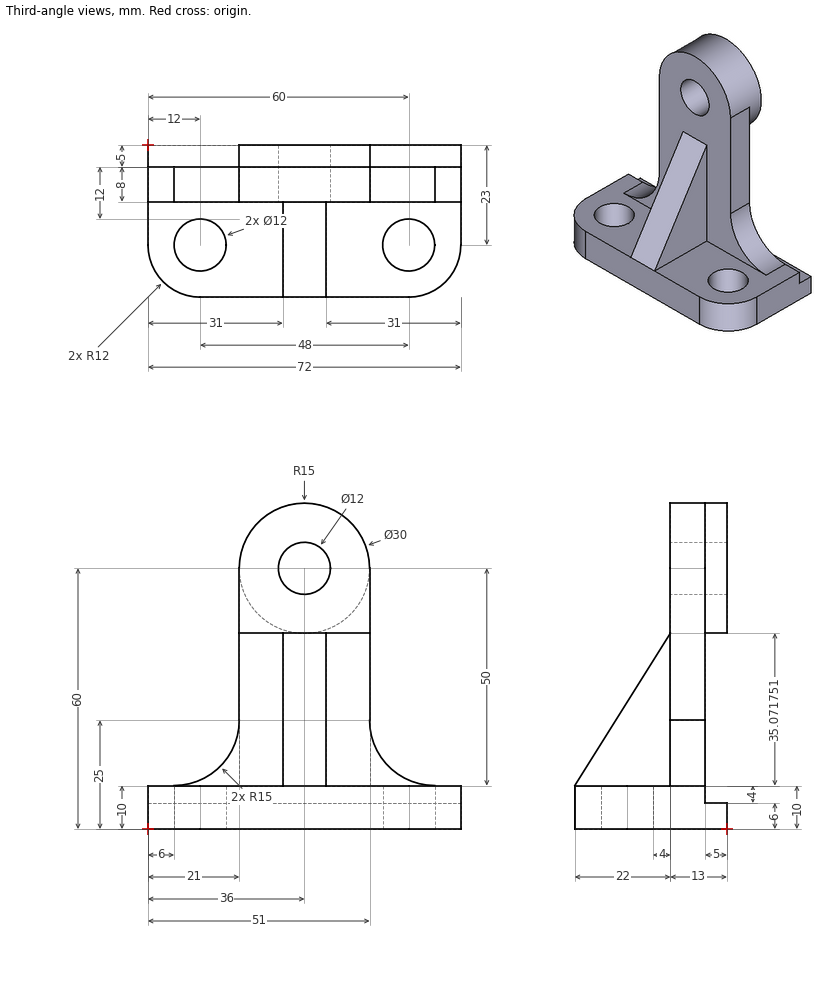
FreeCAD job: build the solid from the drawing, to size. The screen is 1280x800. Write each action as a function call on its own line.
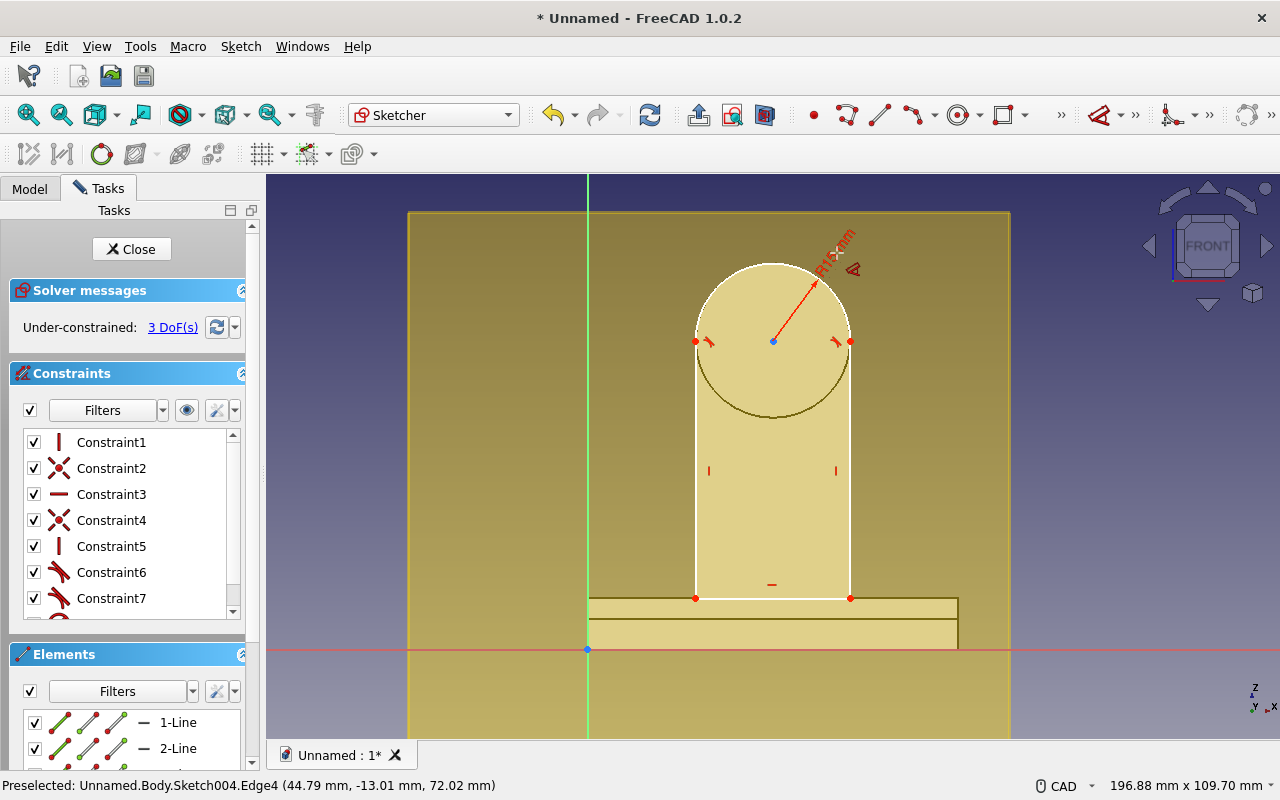
click(696, 418)
click(662, 470)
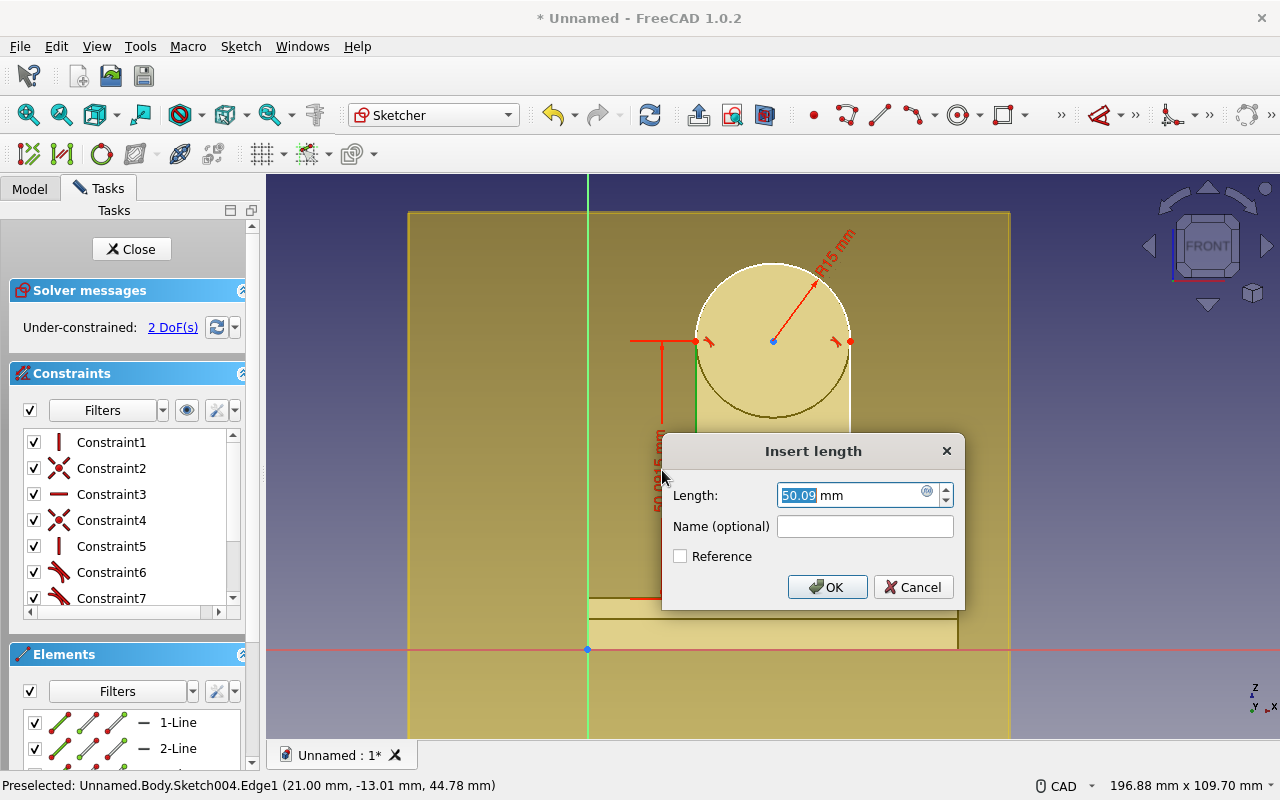
text(50)
key(Return)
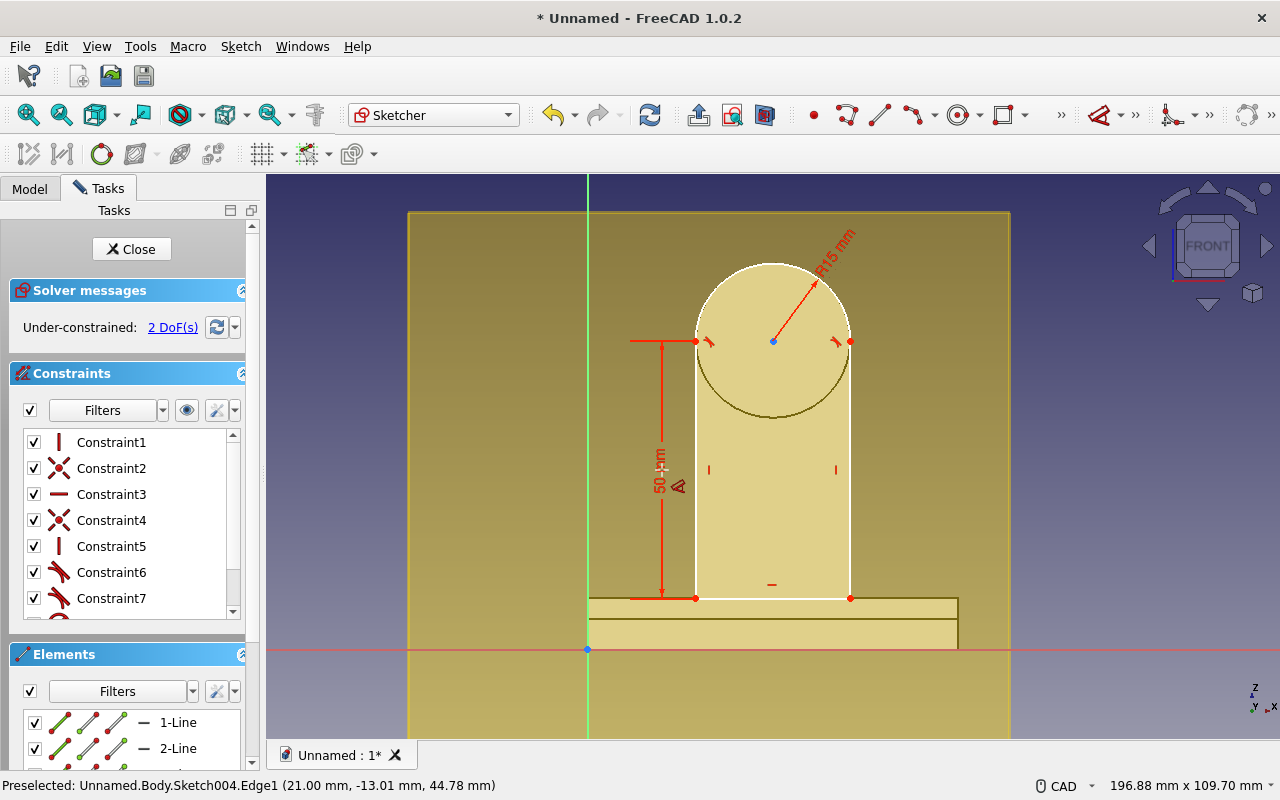
click(696, 341)
click(642, 684)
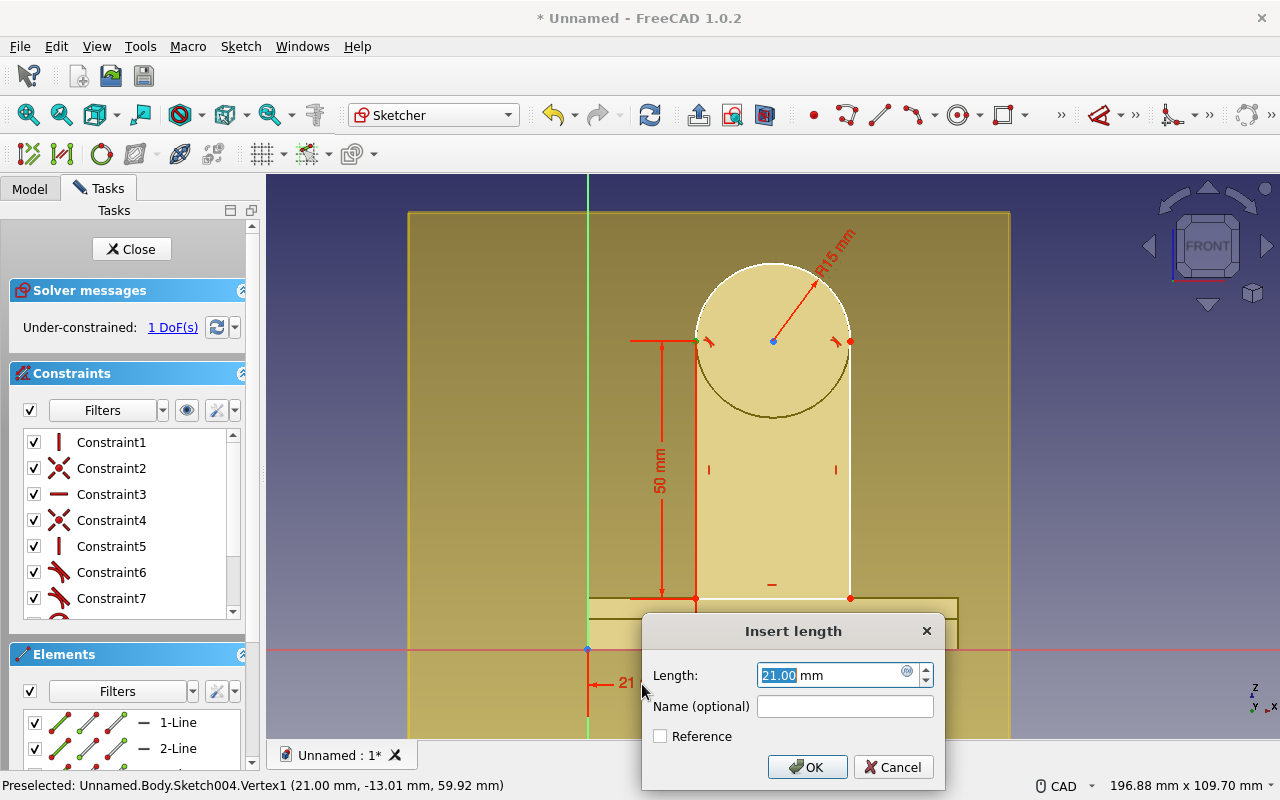
text(21)
key(Return)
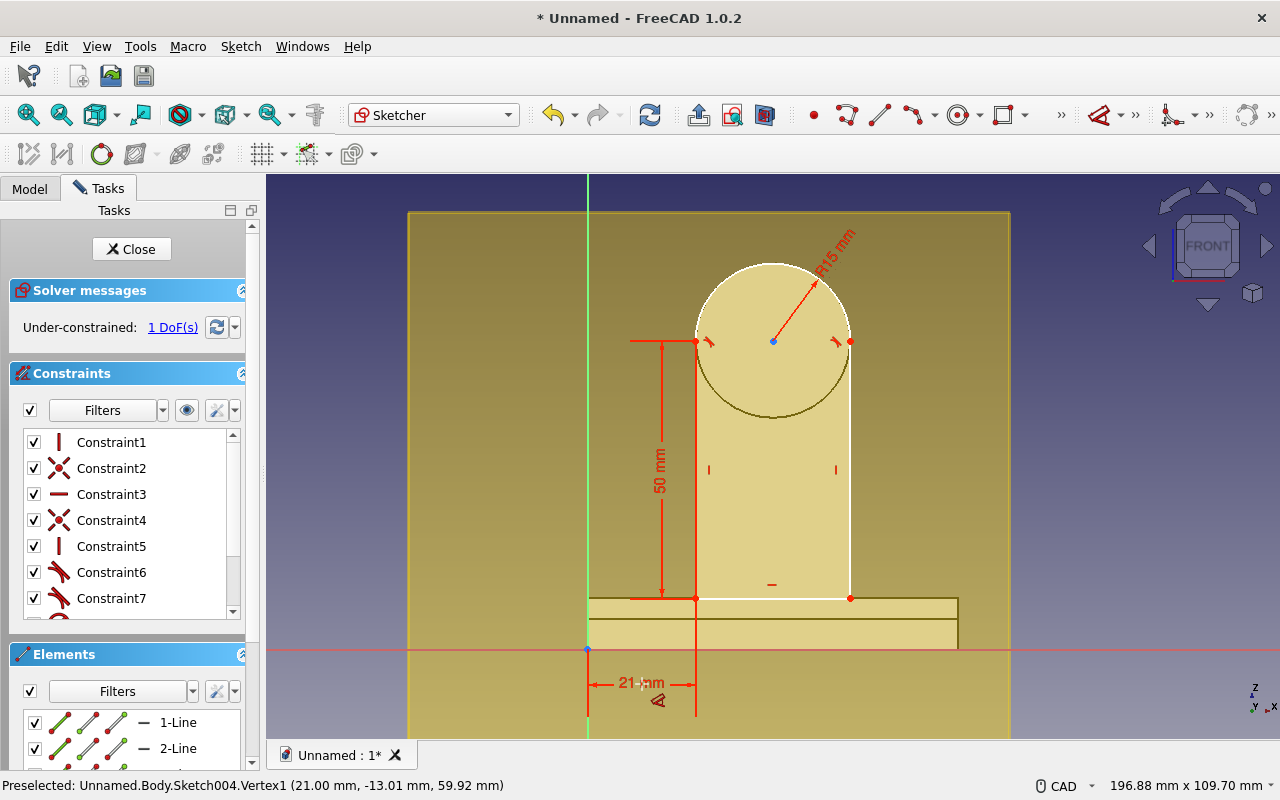
click(696, 341)
click(554, 495)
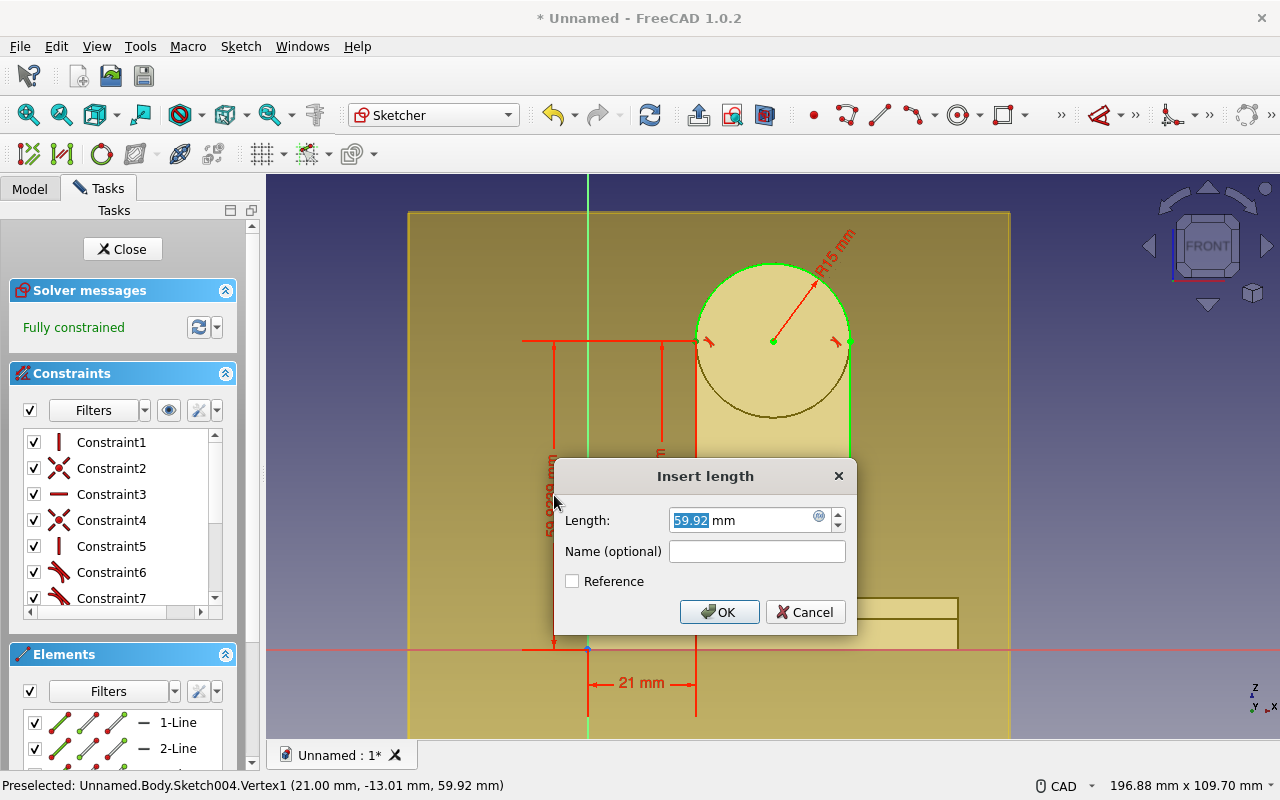
text(60)
key(Return)
key(Escape)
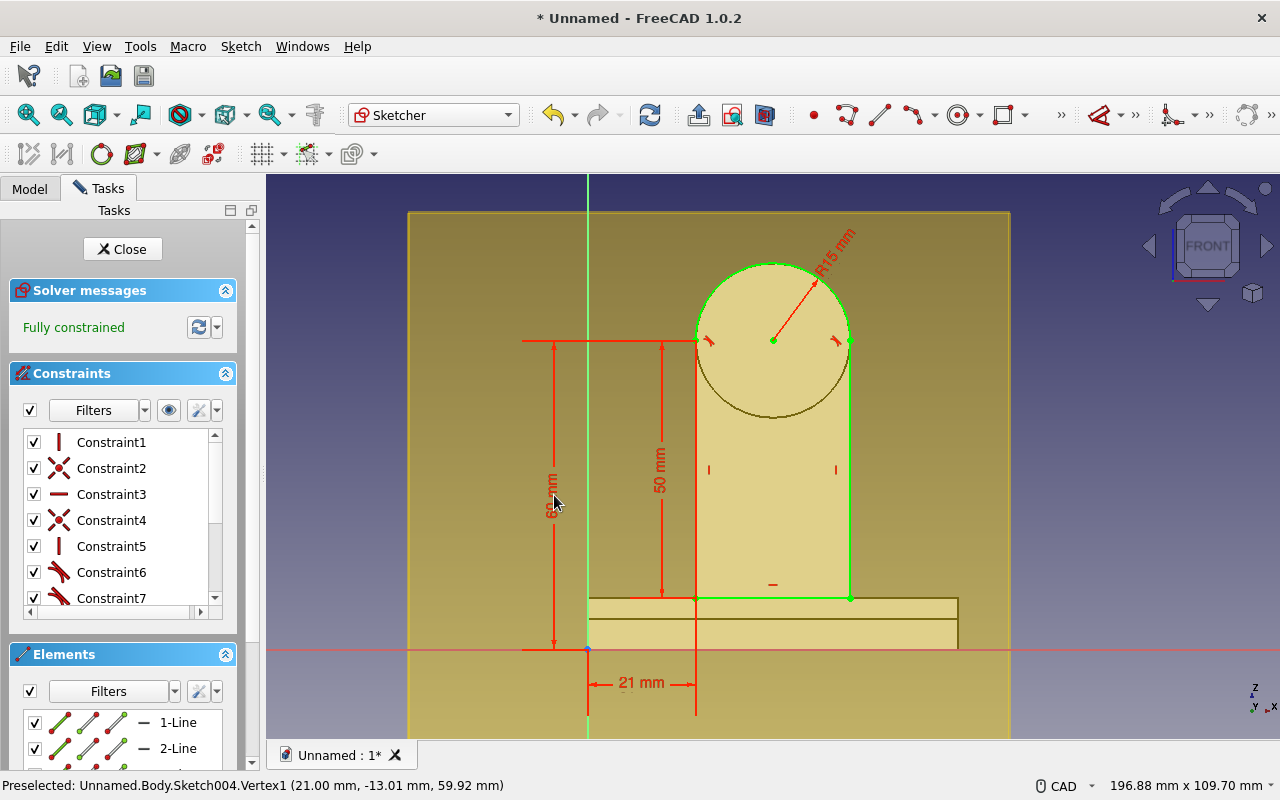
click(123, 249)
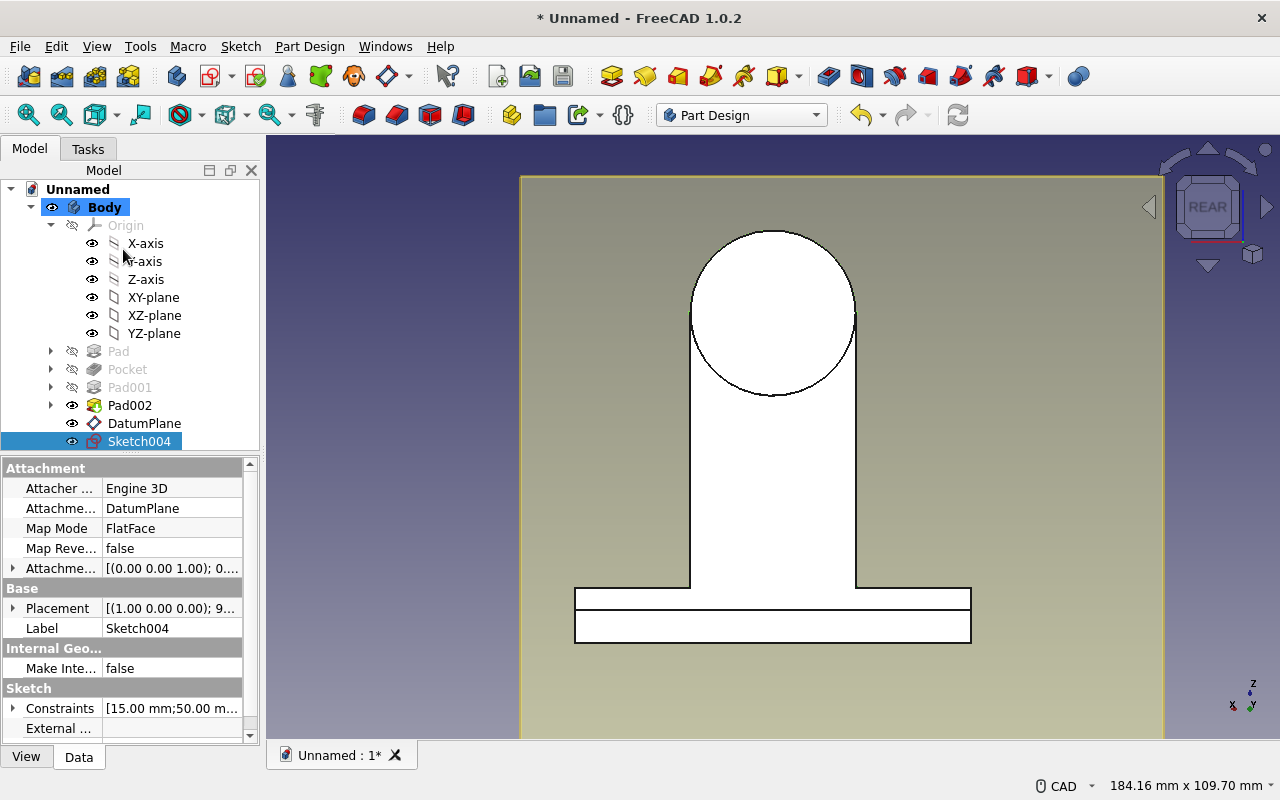
click(829, 76)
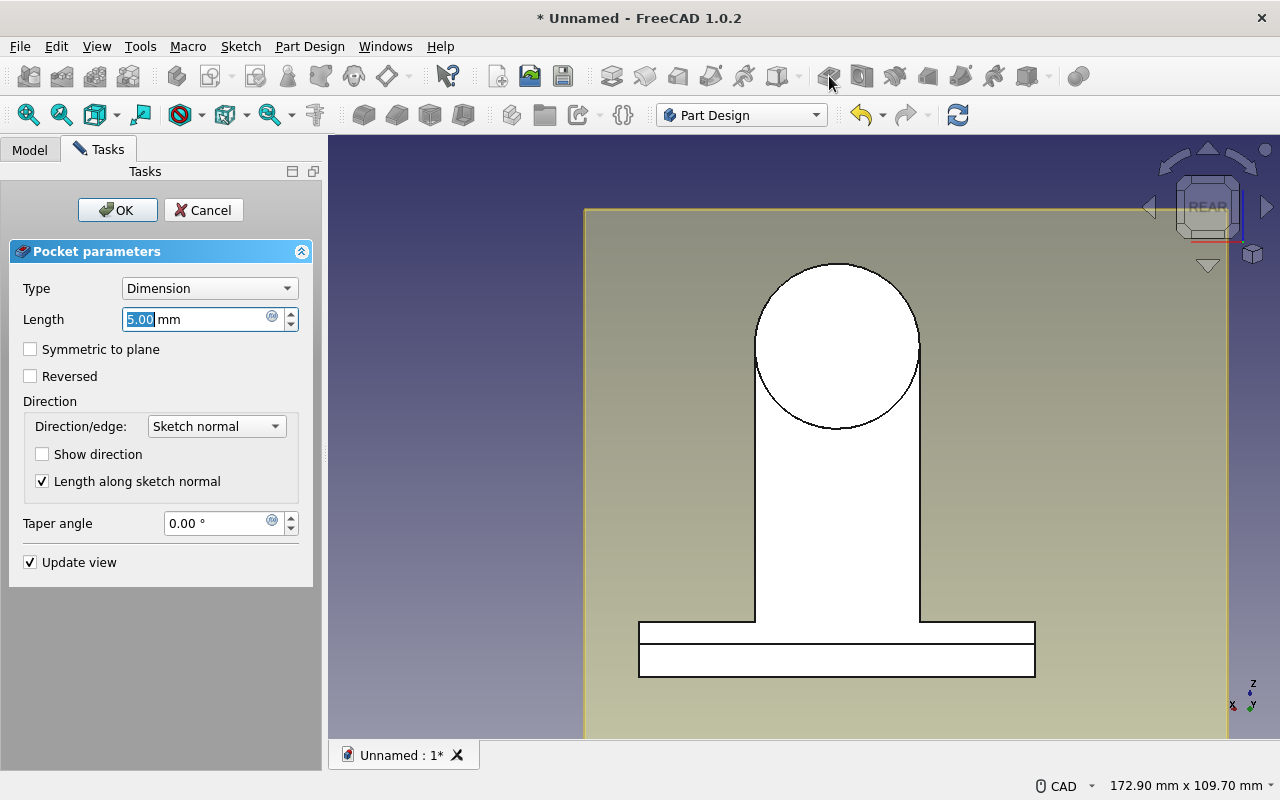
text(4)
key(Tab)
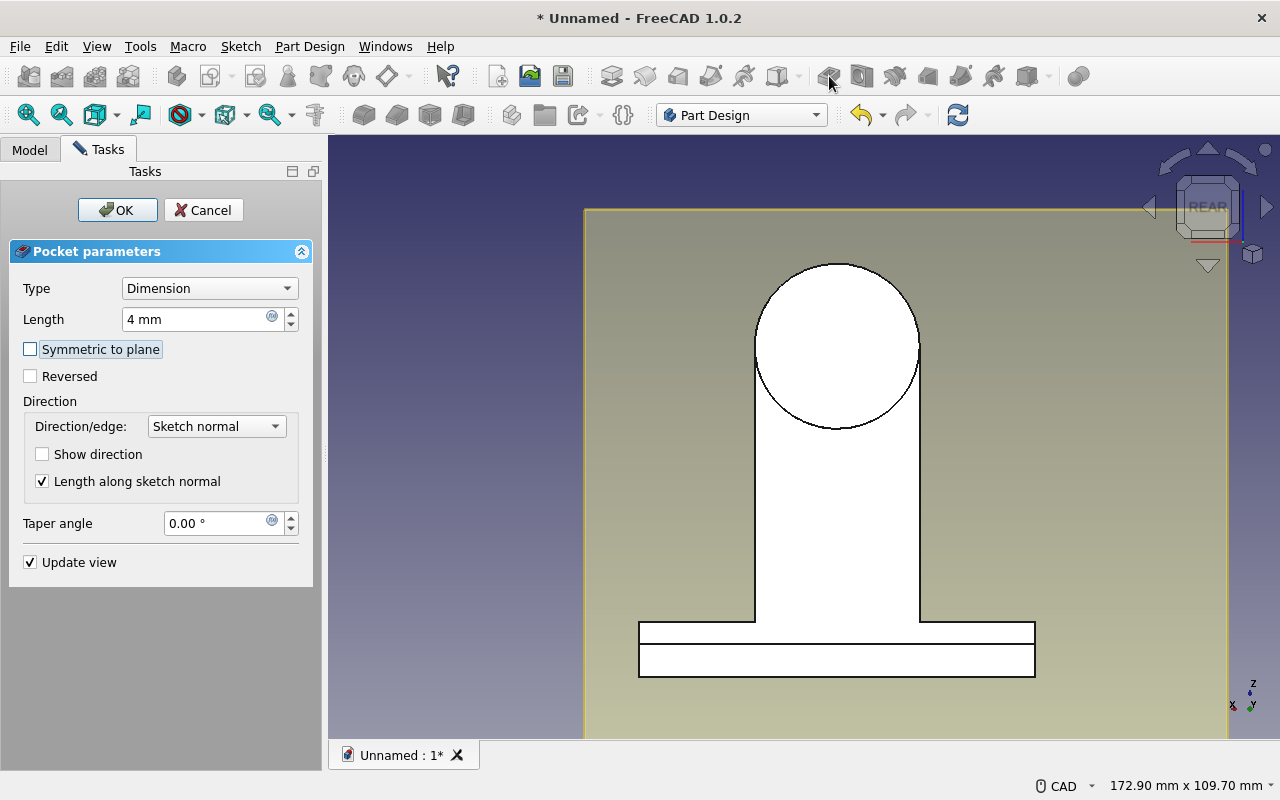
click(31, 376)